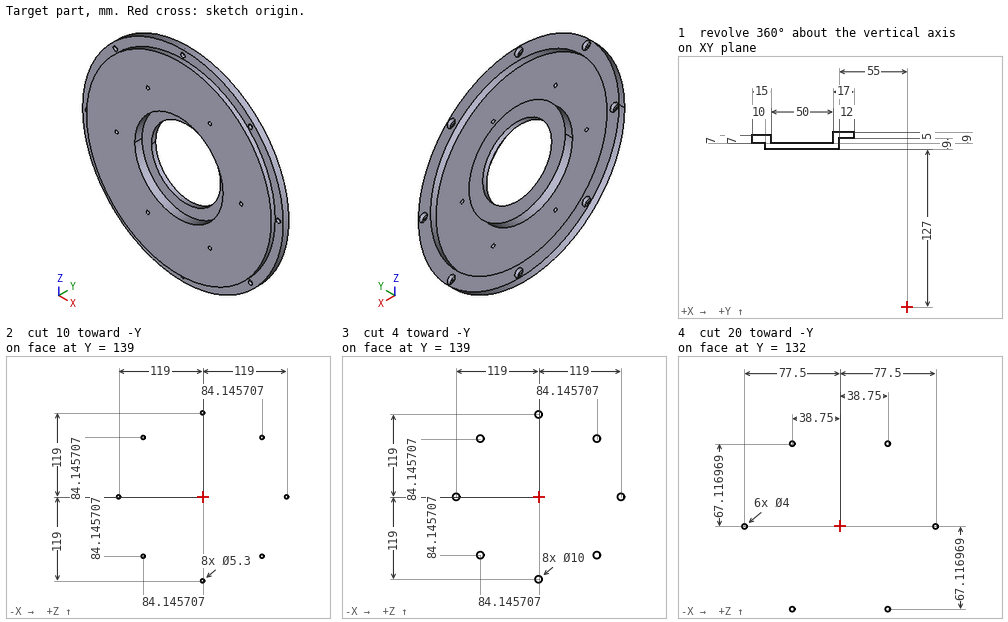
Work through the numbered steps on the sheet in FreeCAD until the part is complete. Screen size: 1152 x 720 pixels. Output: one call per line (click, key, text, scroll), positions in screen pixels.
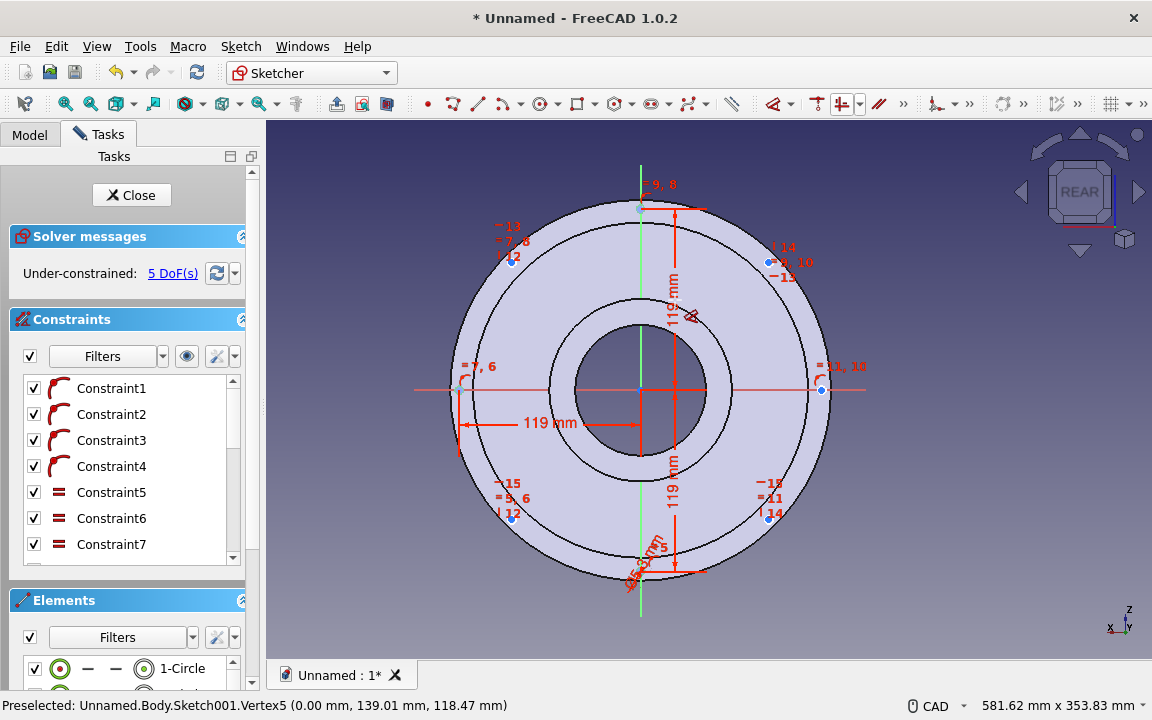
click(822, 390)
click(731, 424)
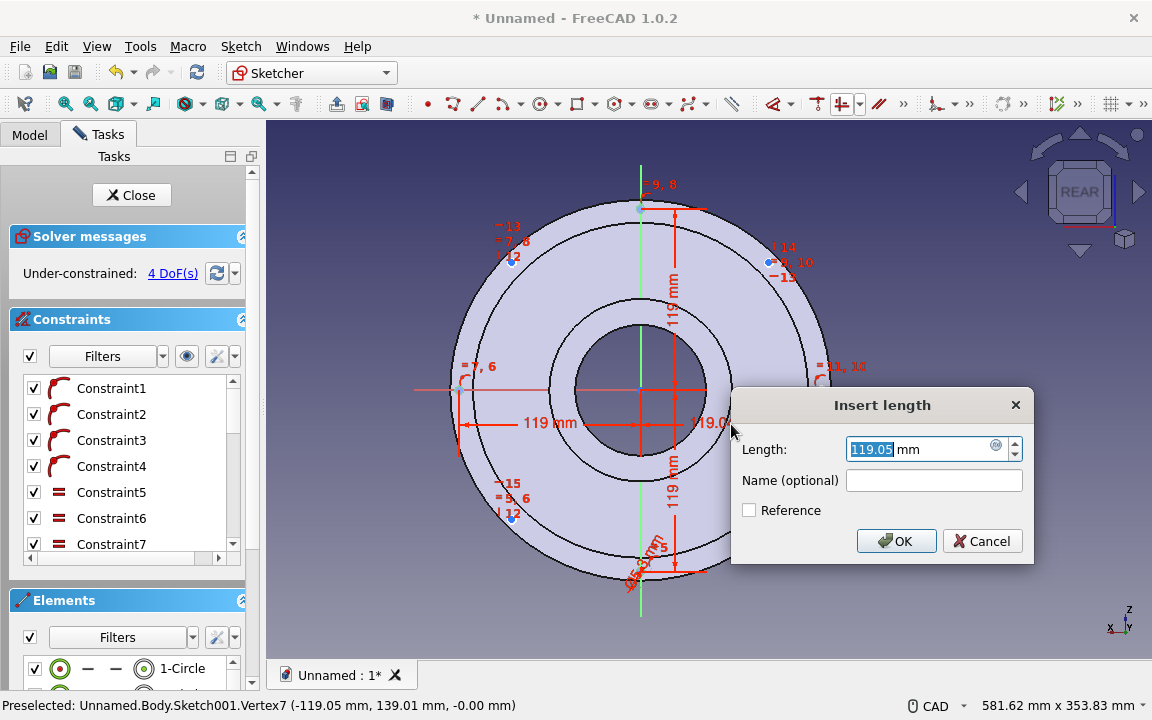
text(119)
key(Return)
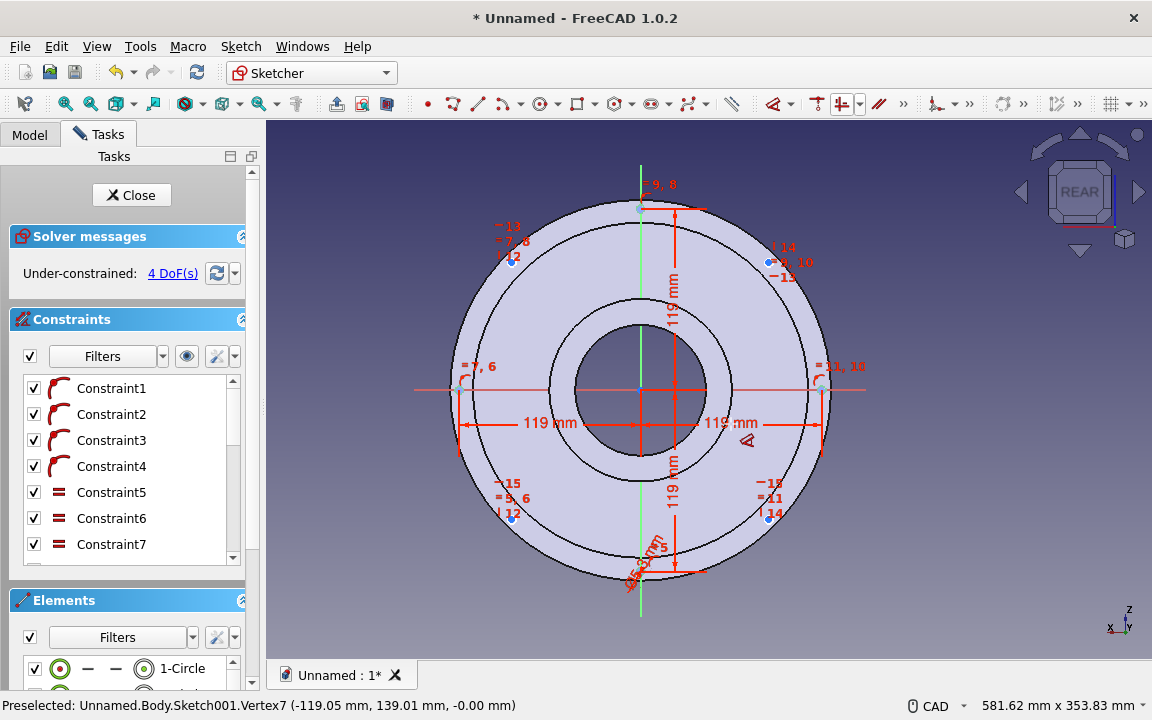
click(512, 520)
click(547, 554)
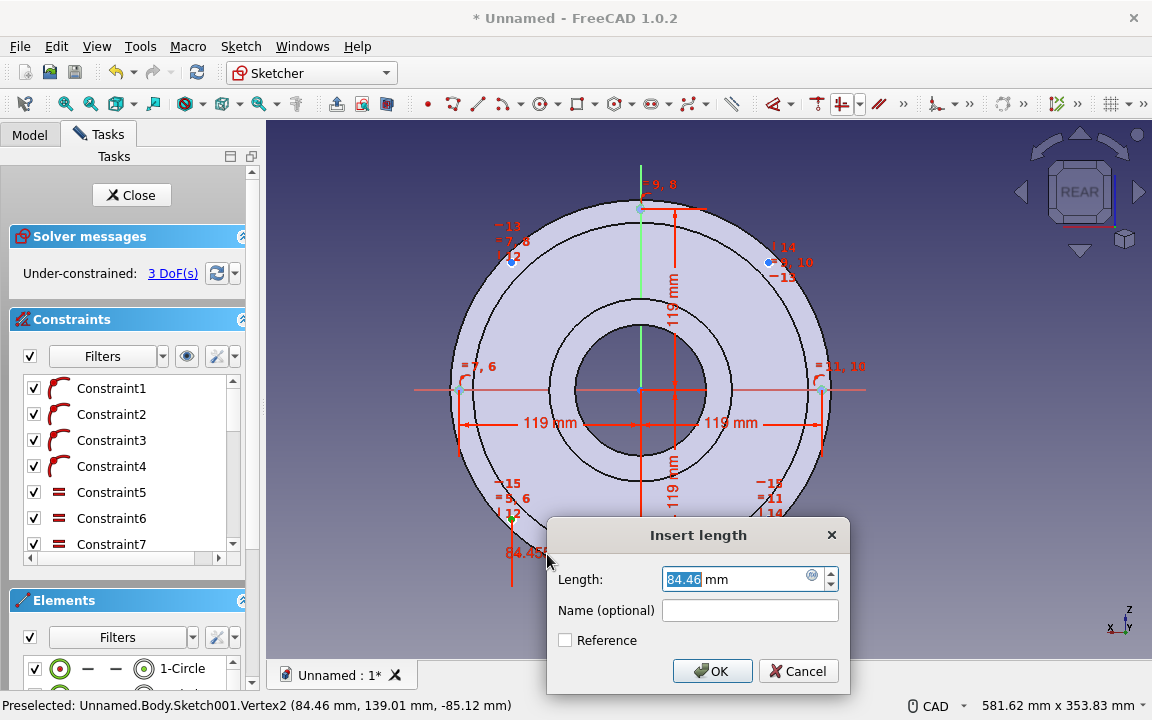
text(84.145707)
key(Return)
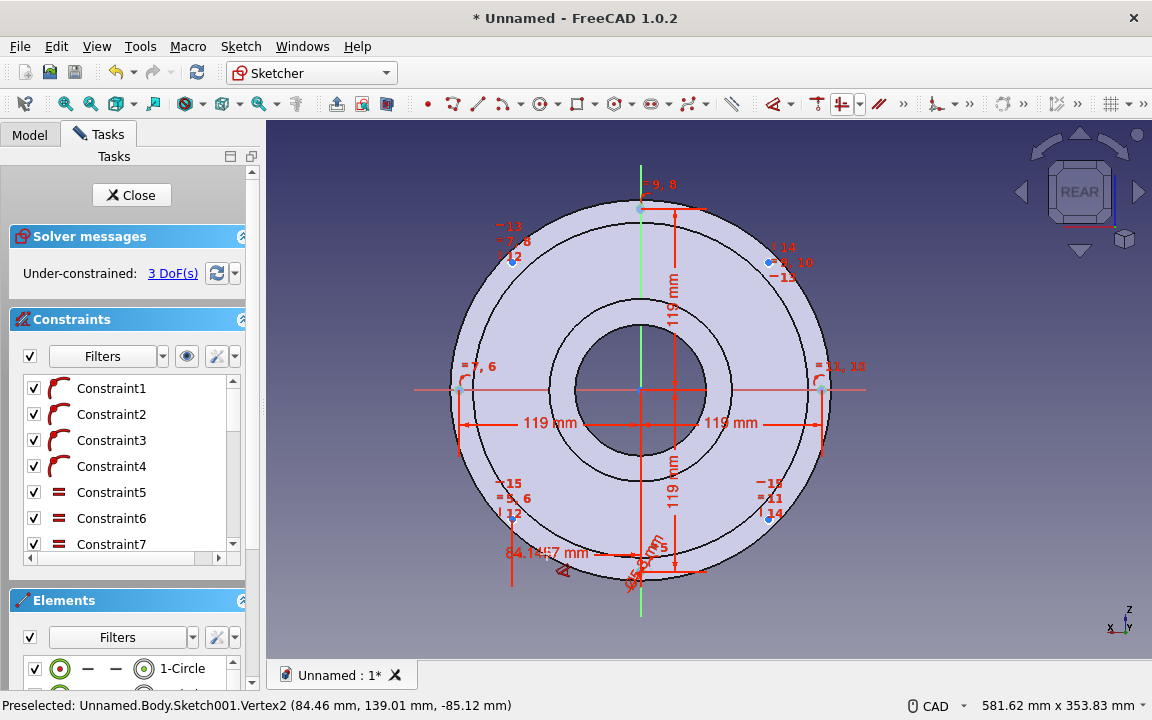
click(512, 520)
click(478, 455)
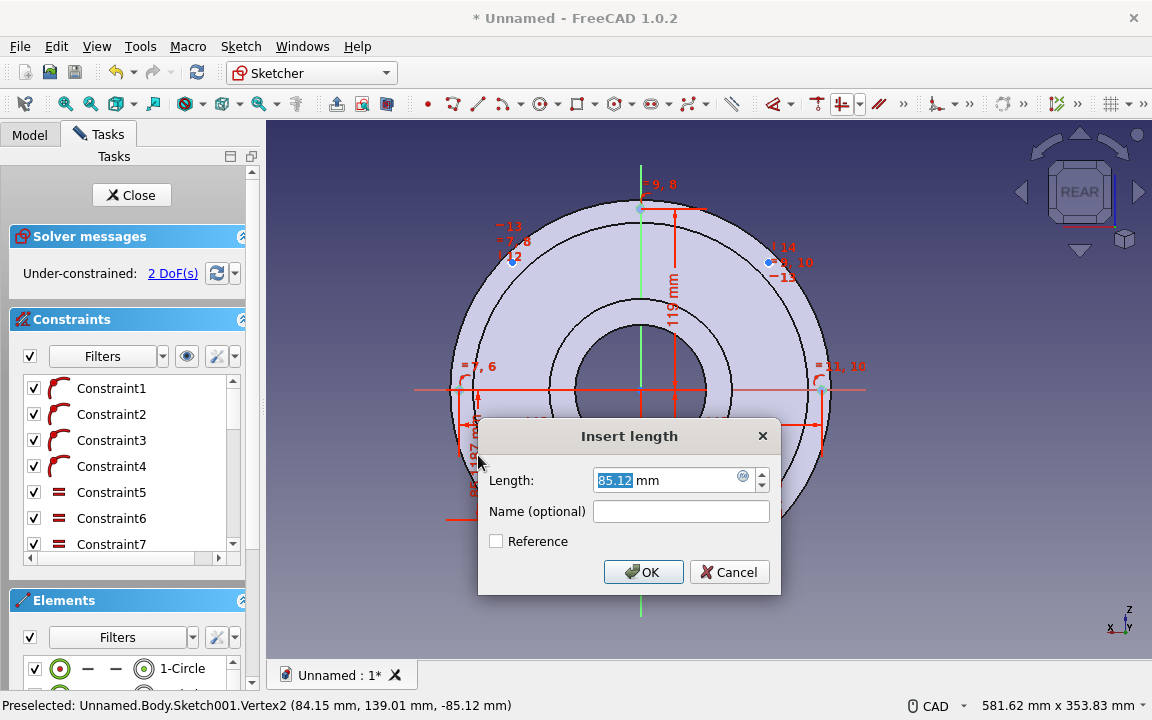
text(84.145707)
key(Return)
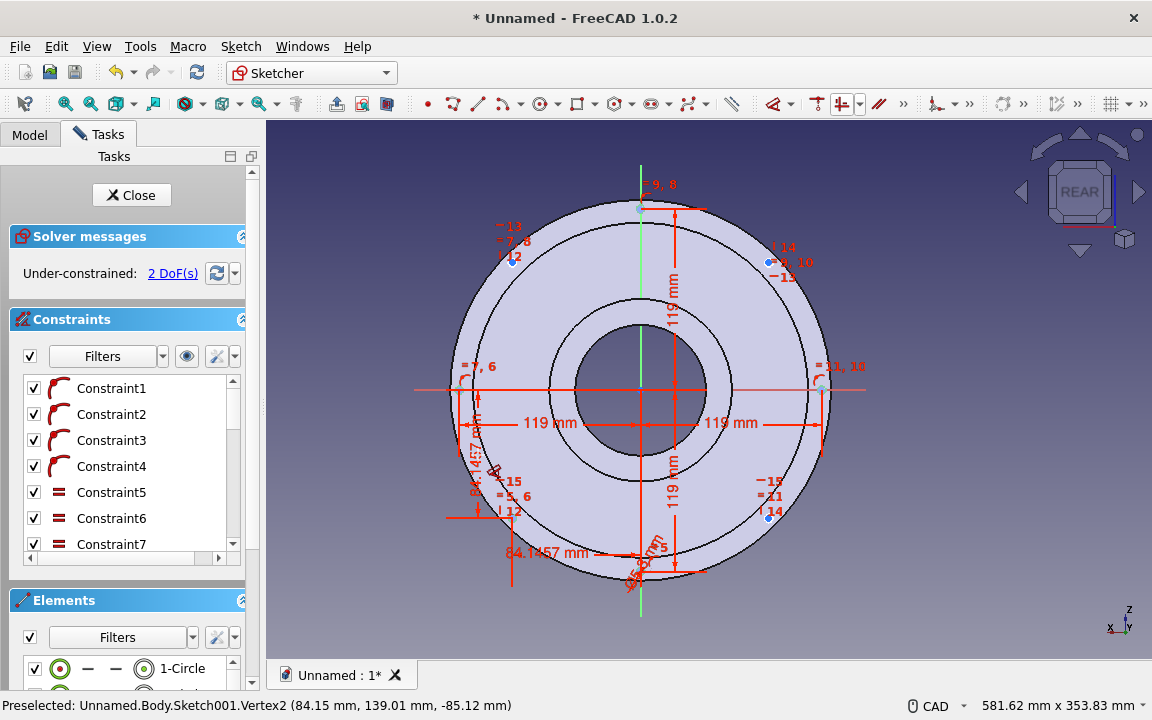
click(512, 263)
click(478, 327)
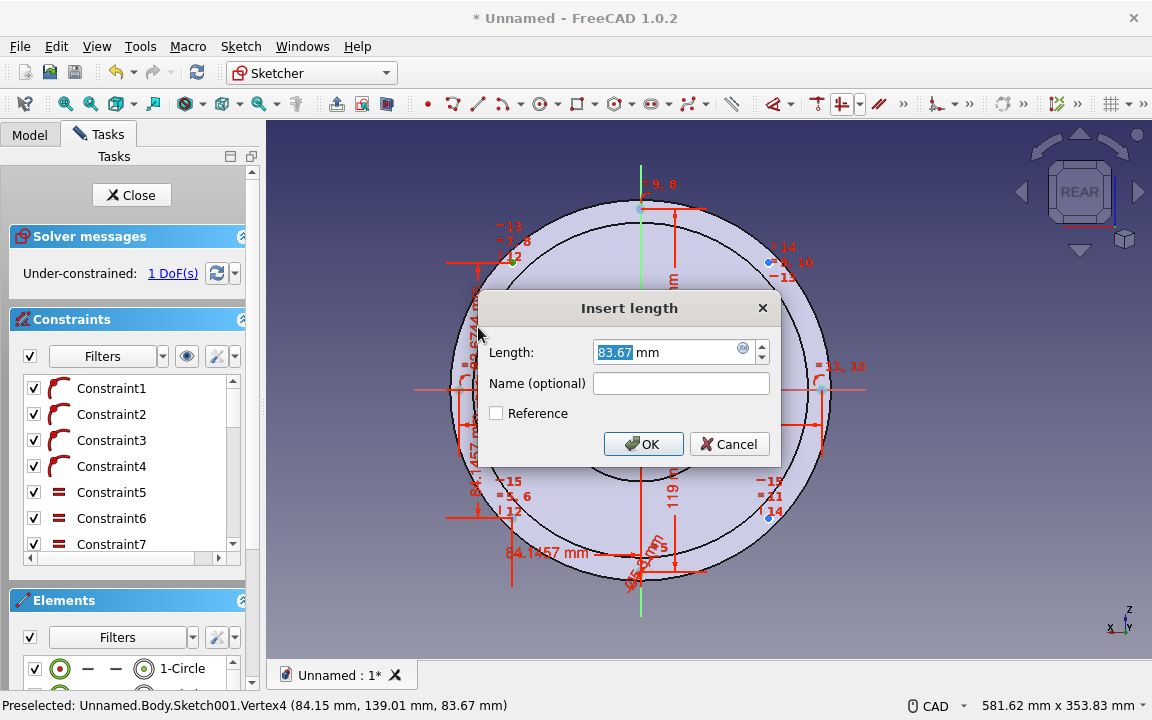
text(84.145707)
key(Return)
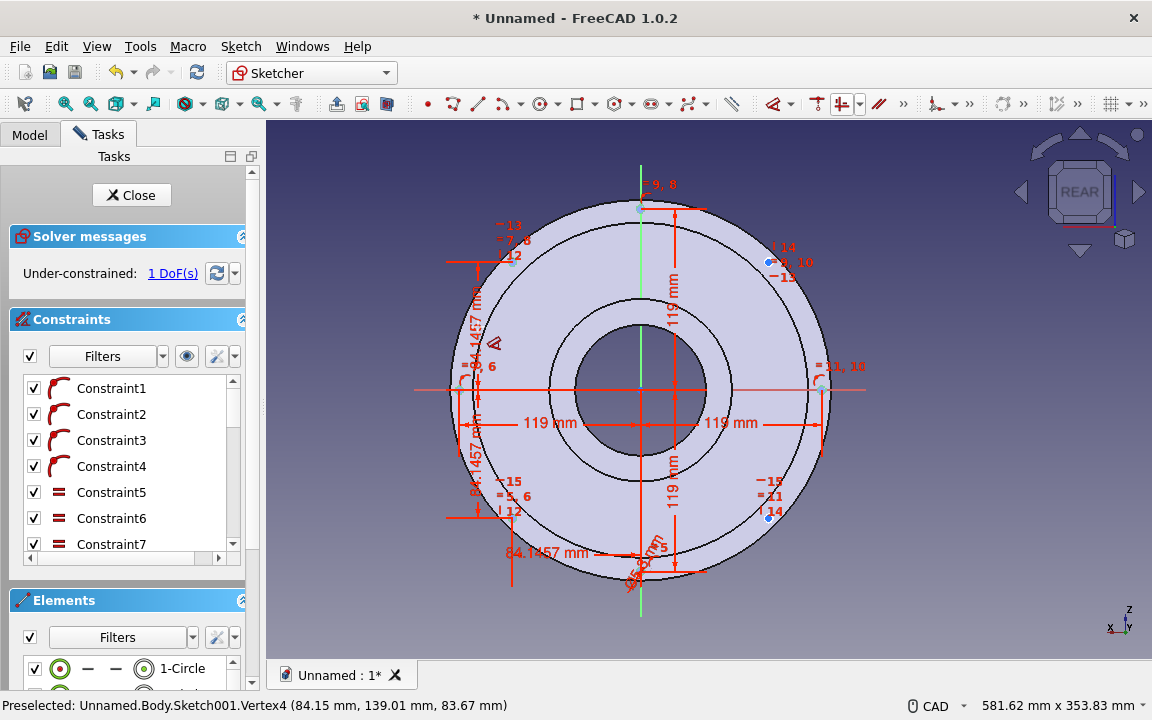
click(769, 262)
click(705, 228)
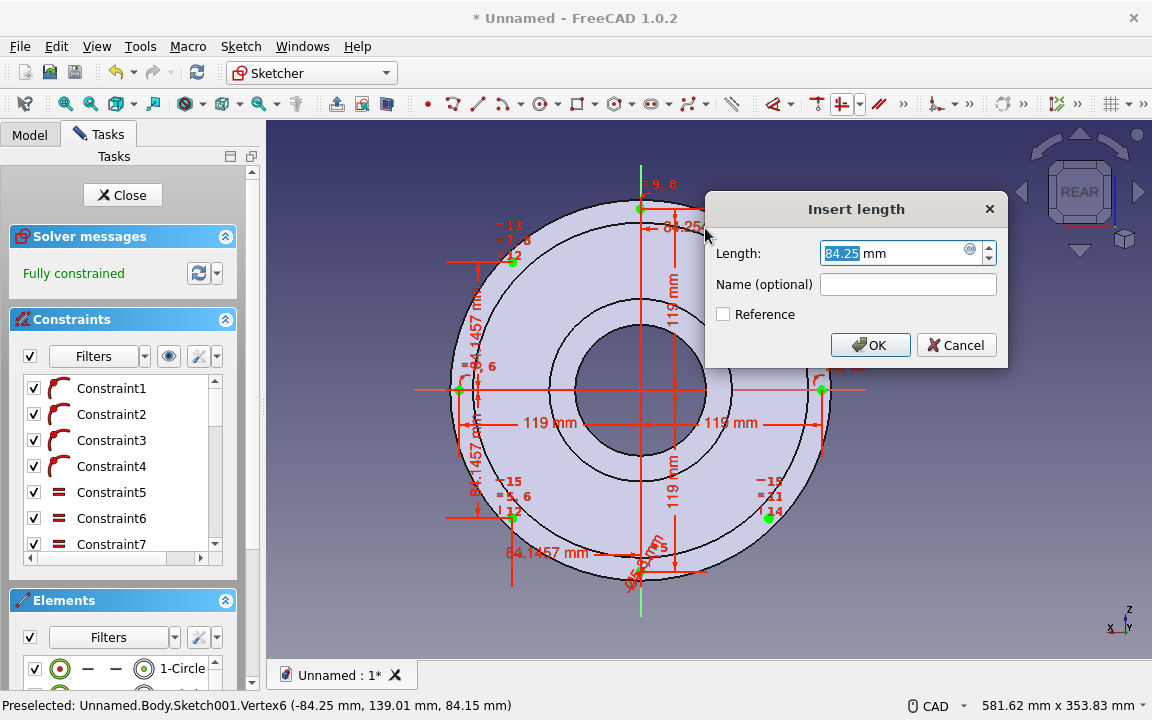
text(84.145707)
key(Return)
key(Escape)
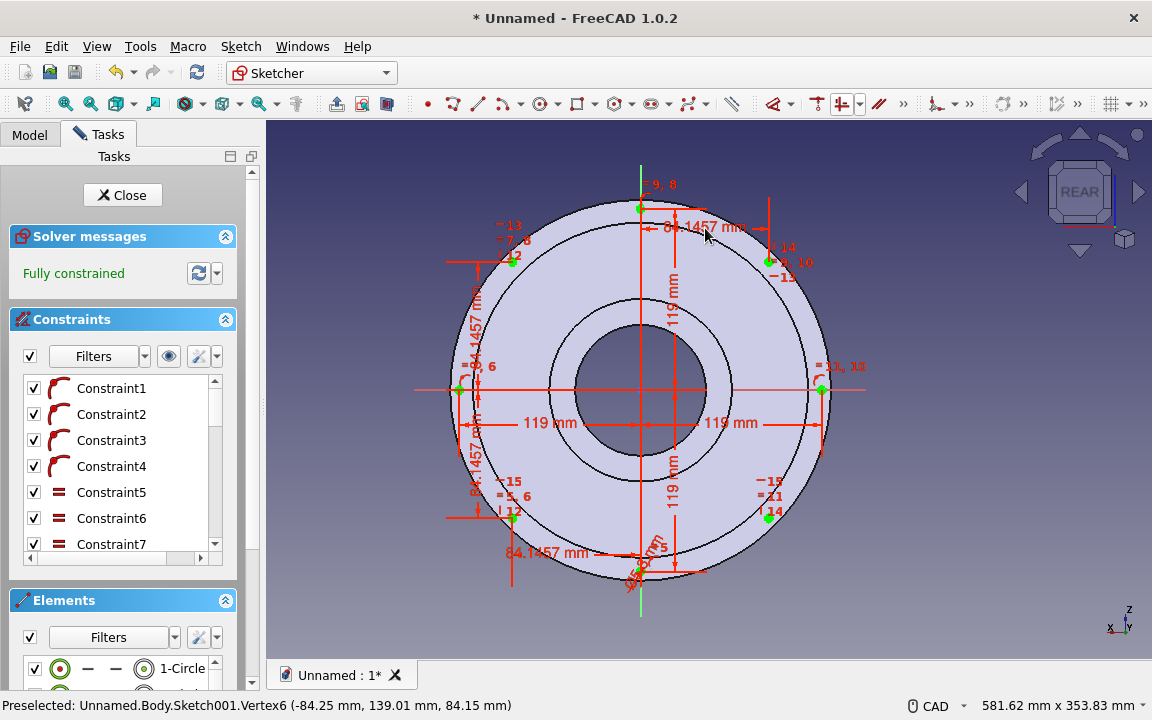
click(123, 195)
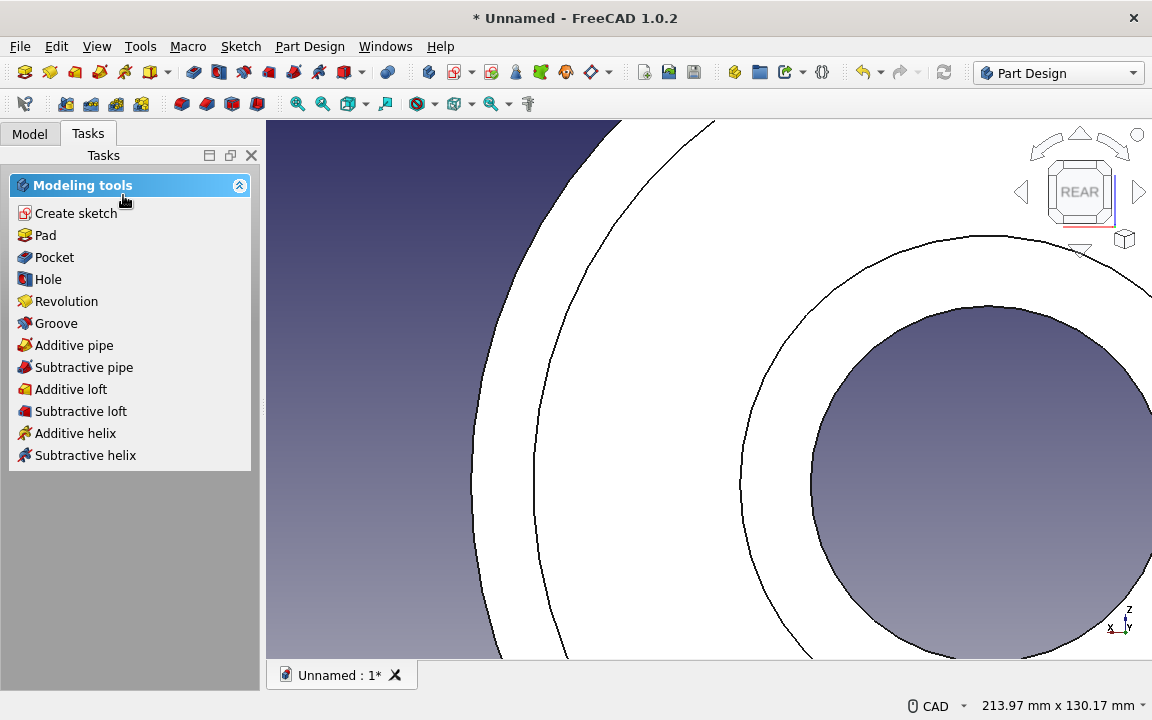
click(194, 72)